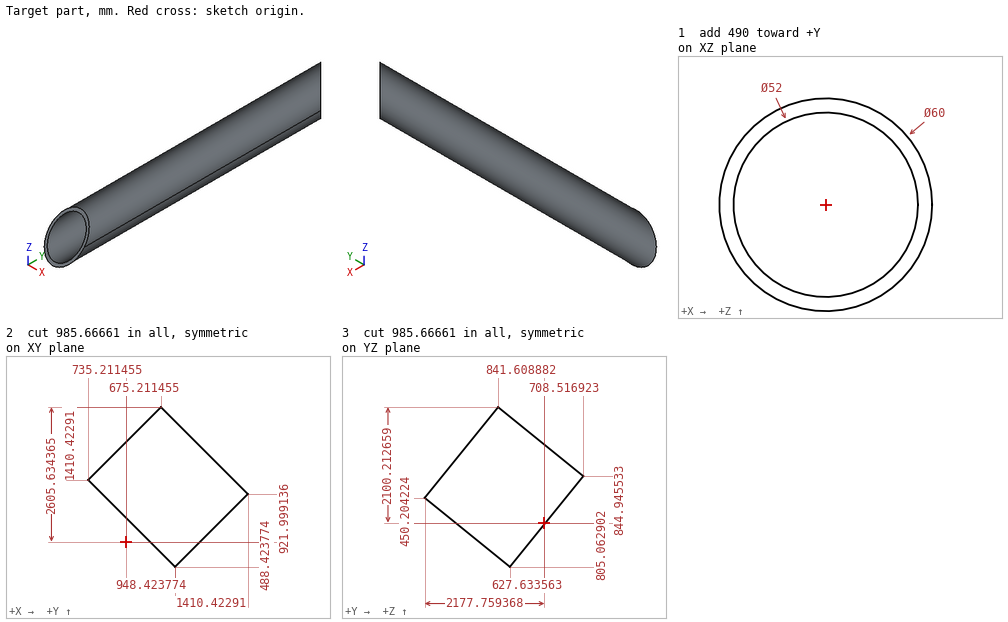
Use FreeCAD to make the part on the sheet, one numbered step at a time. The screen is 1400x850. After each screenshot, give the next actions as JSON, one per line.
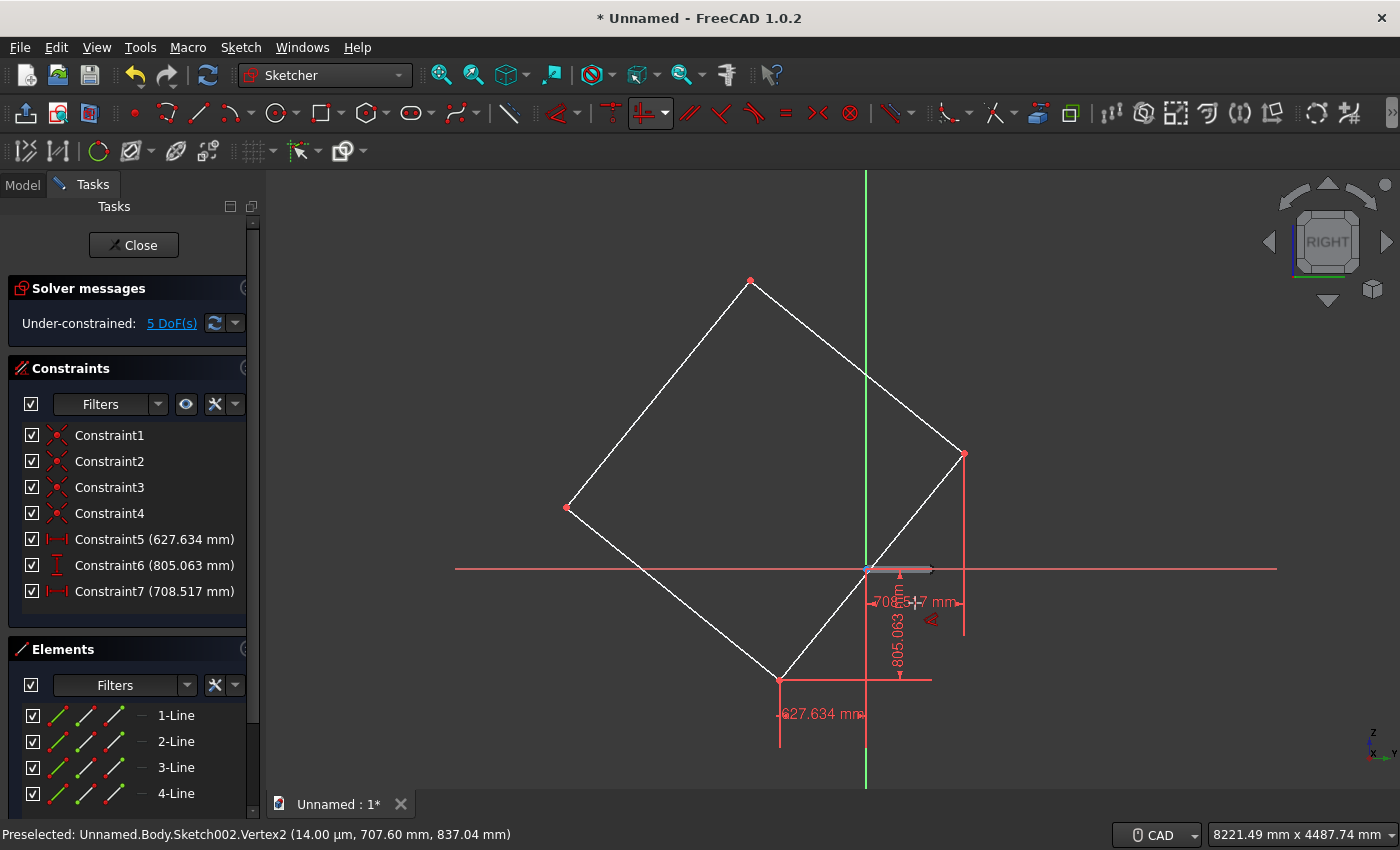
{"action": "left_click", "coordinate": [964, 454]}
{"action": "left_click", "coordinate": [998, 512]}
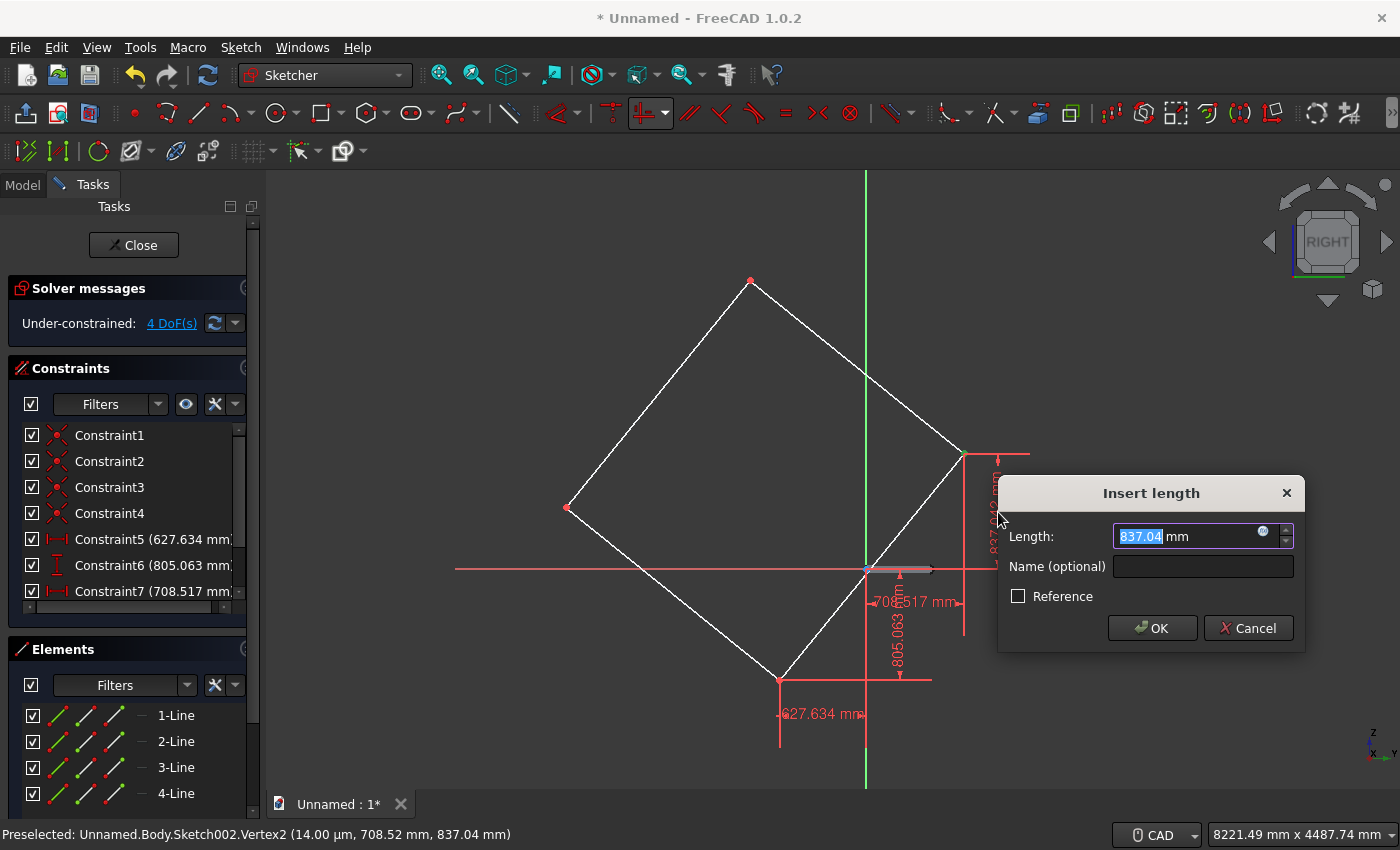
{"action": "type", "text": "844.945533"}
{"action": "key", "text": "Return"}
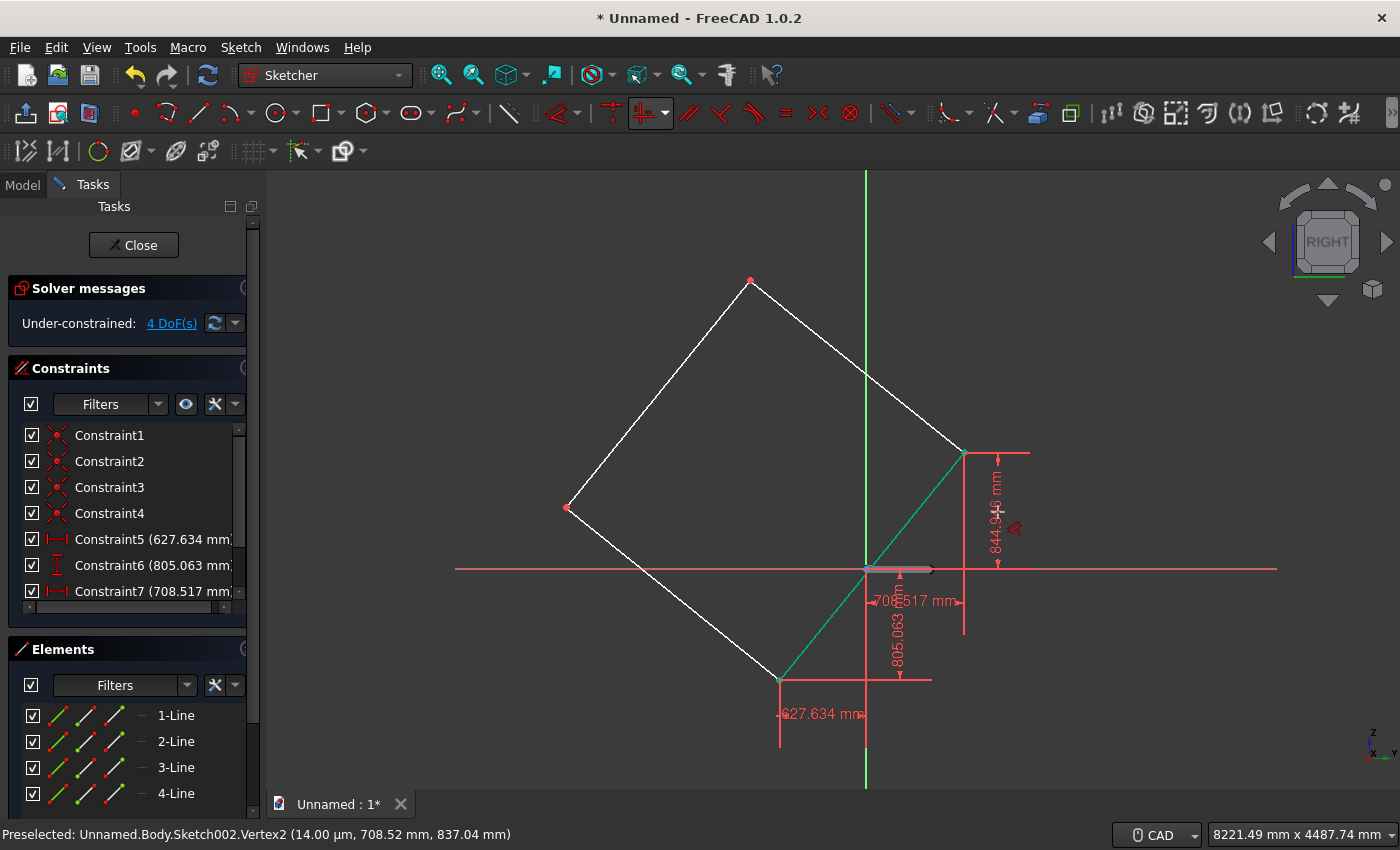
{"action": "left_click", "coordinate": [750, 281]}
{"action": "left_click", "coordinate": [808, 247]}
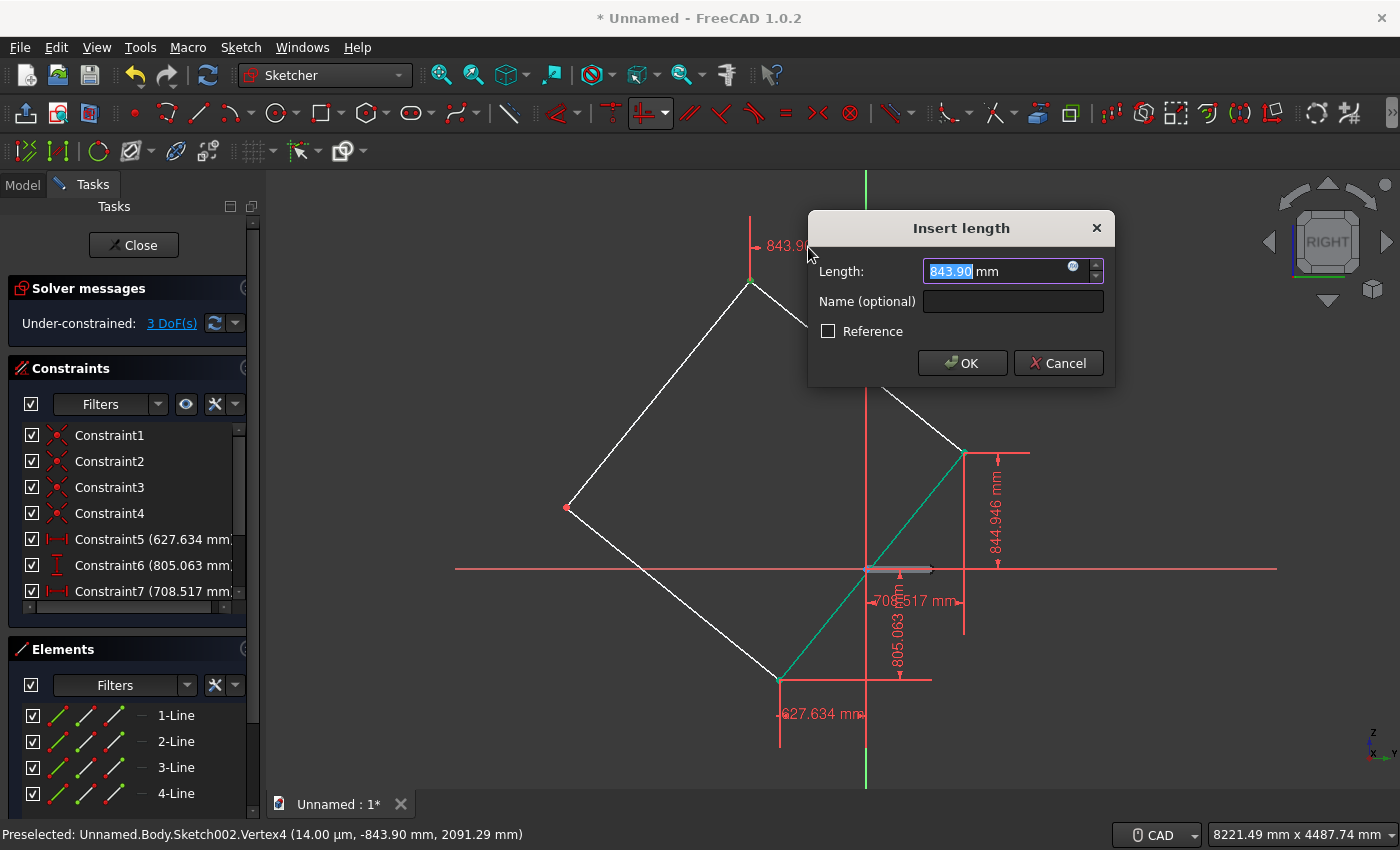
{"action": "type", "text": "841.608882"}
{"action": "key", "text": "Return"}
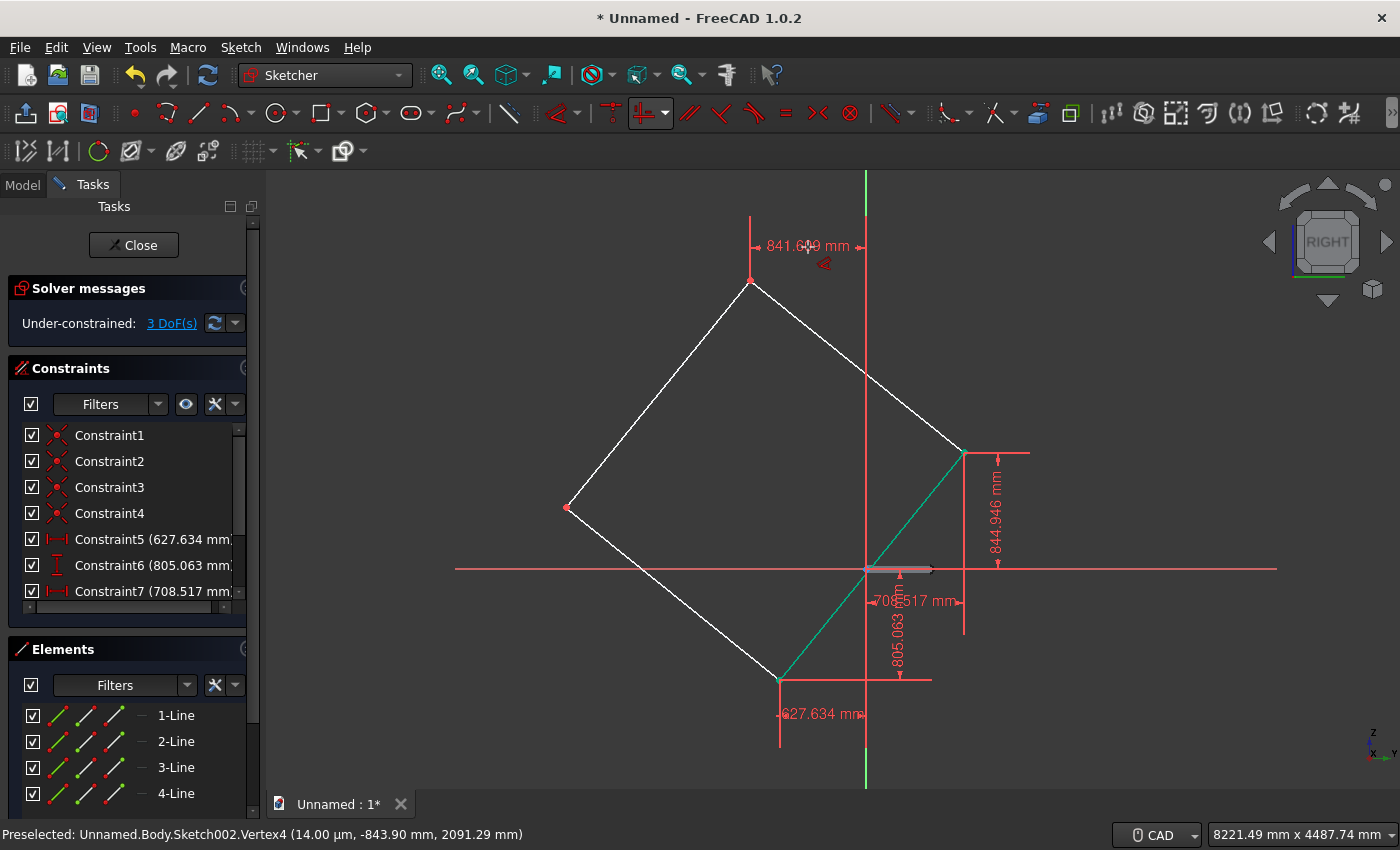
{"action": "left_click", "coordinate": [566, 508]}
{"action": "left_click", "coordinate": [532, 539]}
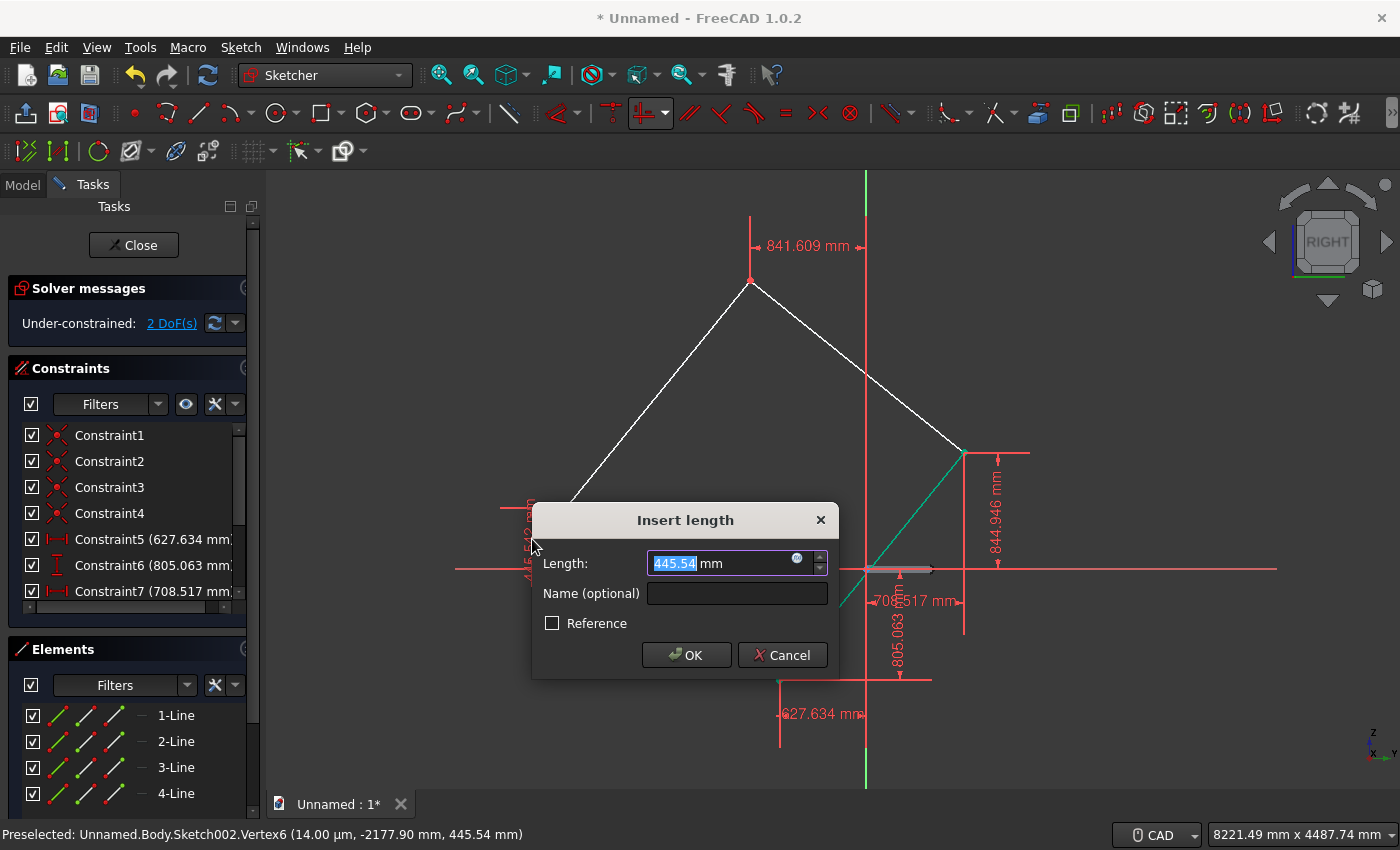
{"action": "type", "text": "450.204224"}
{"action": "key", "text": "Return"}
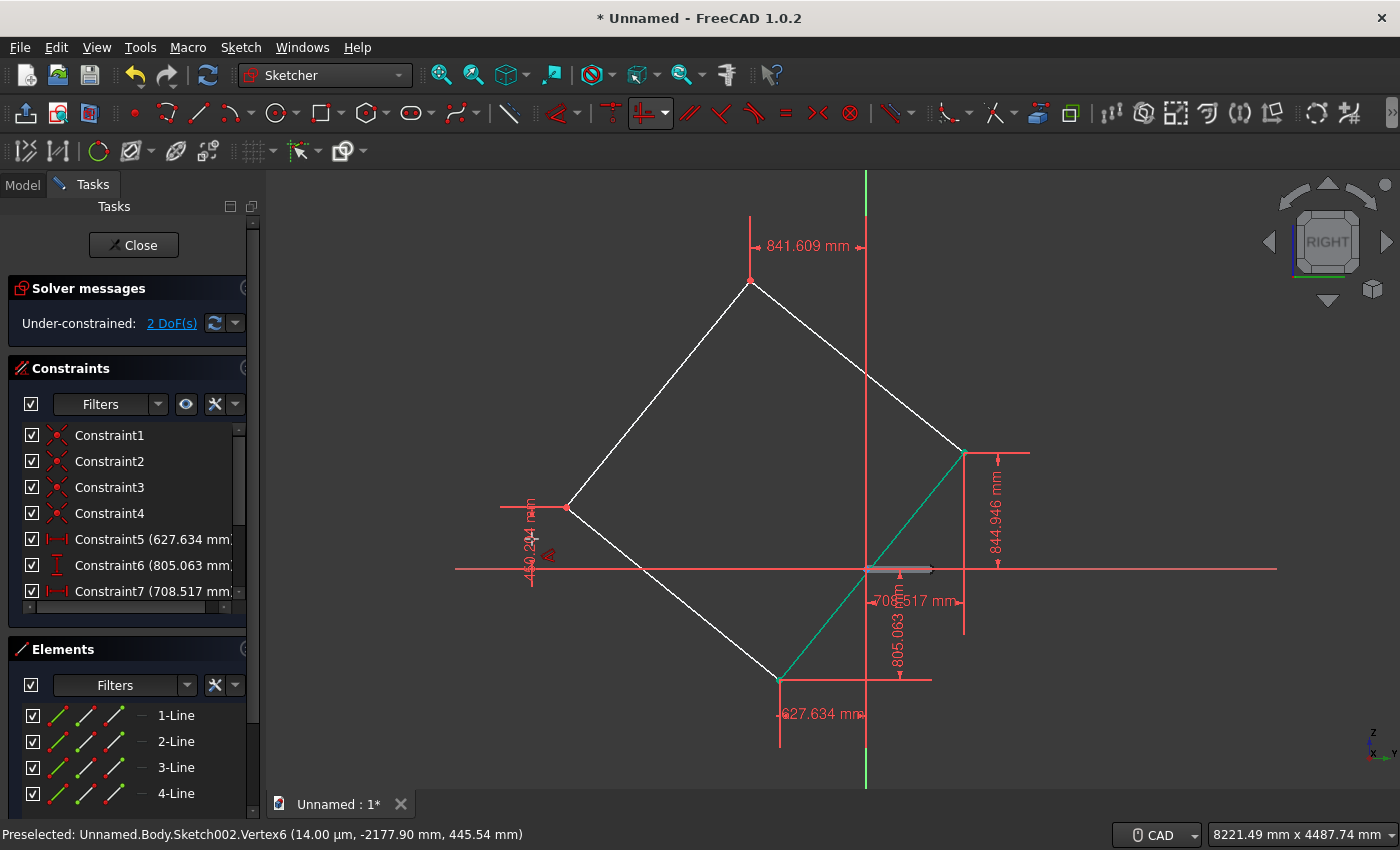
{"action": "left_click", "coordinate": [750, 281]}
{"action": "left_click", "coordinate": [900, 425]}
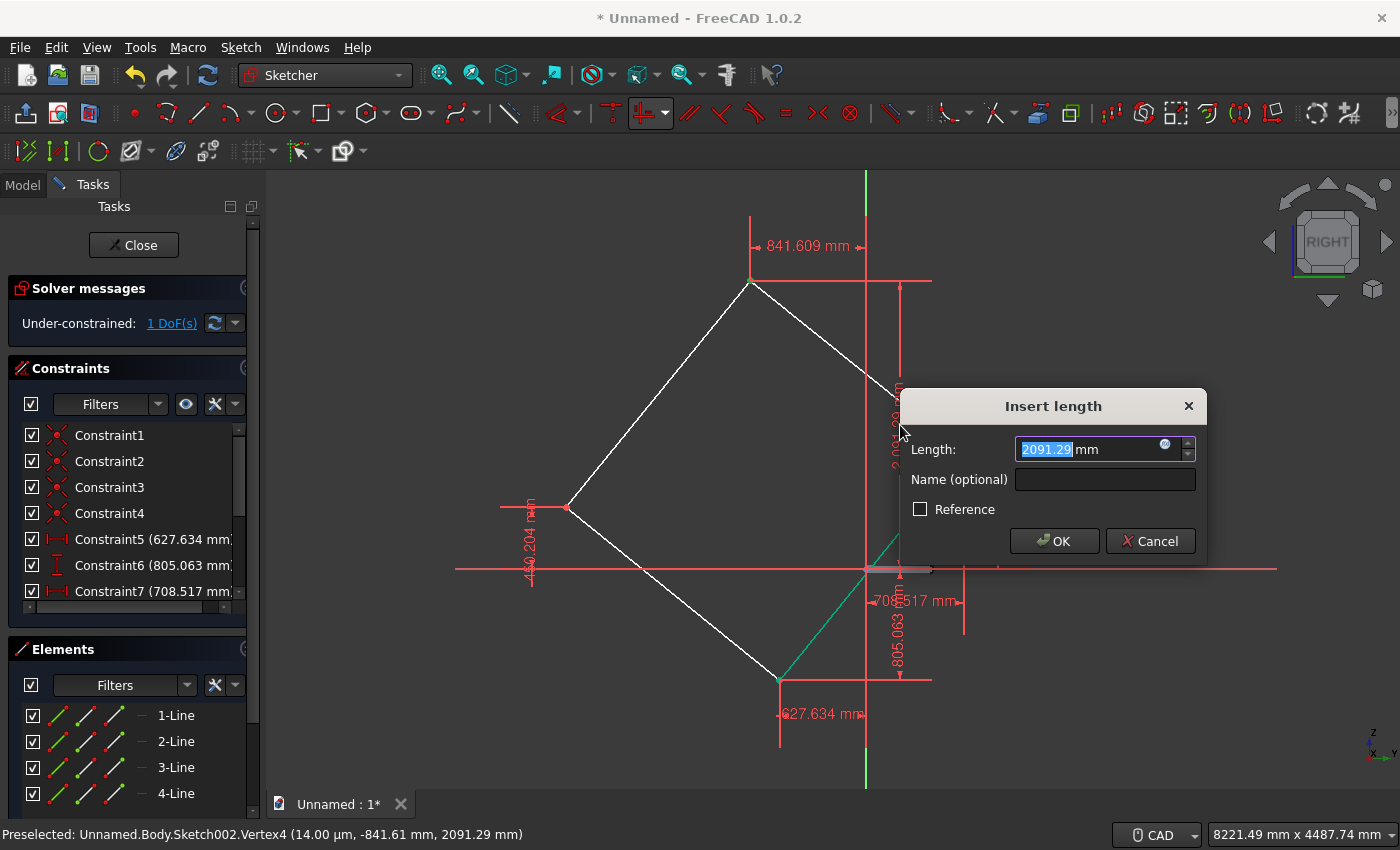
{"action": "type", "text": "2100.212659"}
{"action": "key", "text": "Return"}